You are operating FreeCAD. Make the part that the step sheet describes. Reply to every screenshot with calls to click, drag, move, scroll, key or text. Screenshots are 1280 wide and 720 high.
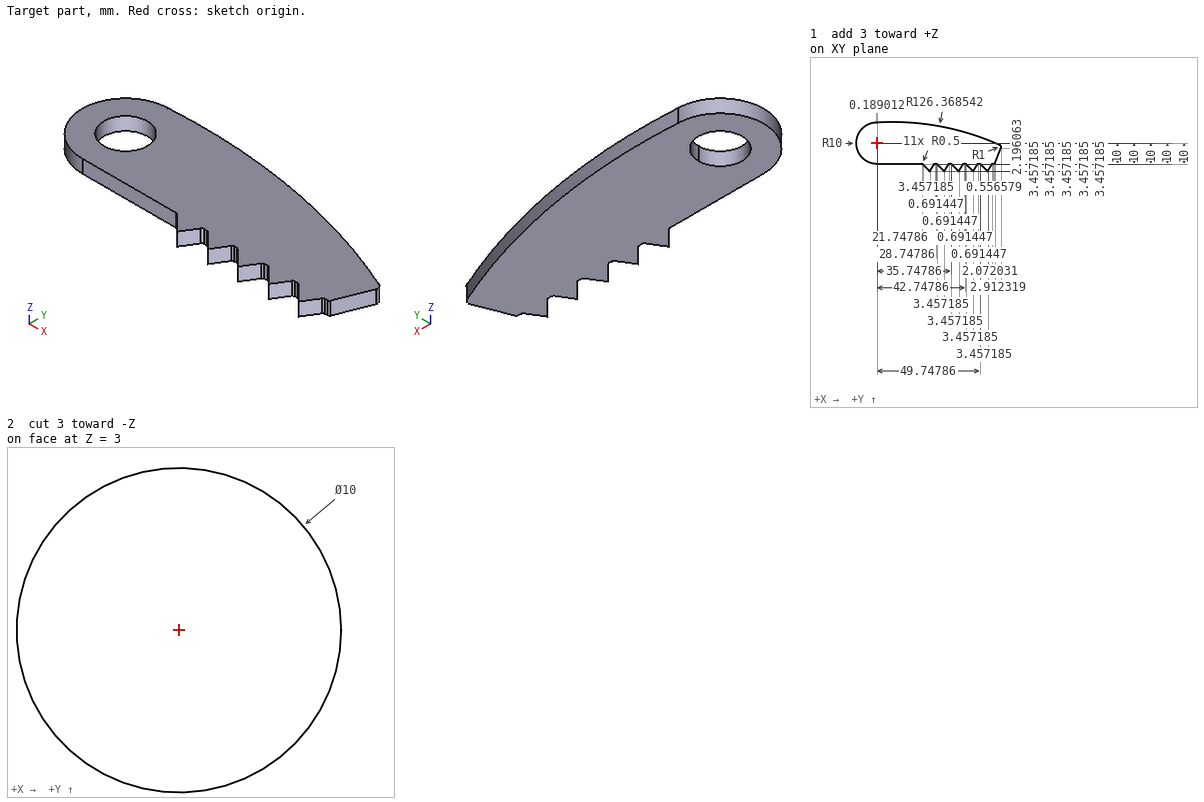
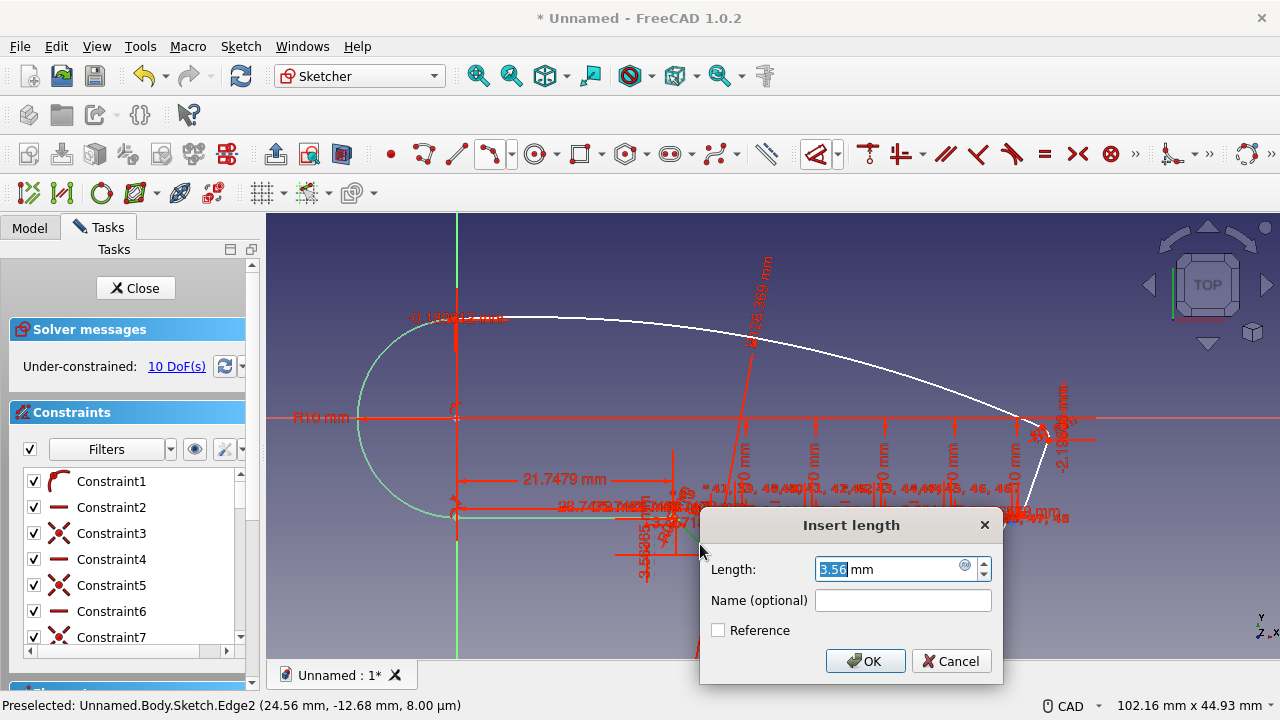
text(3.457185)
key(Return)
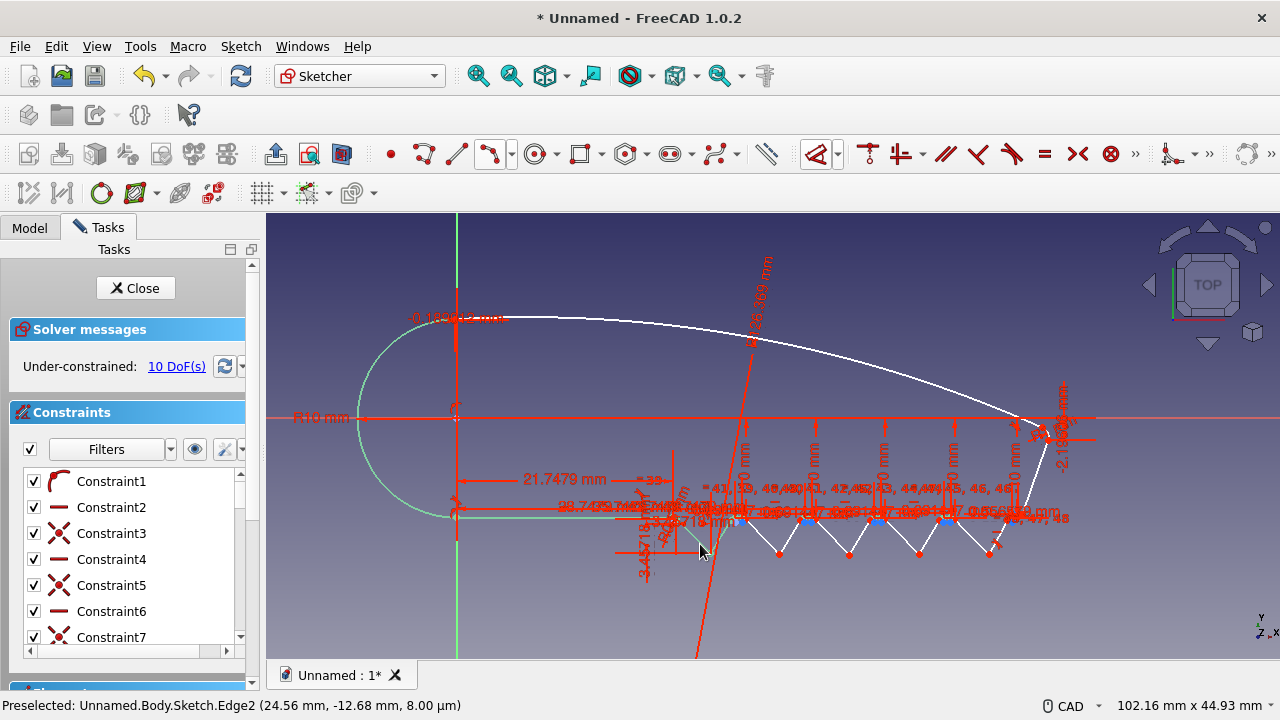
click(756, 530)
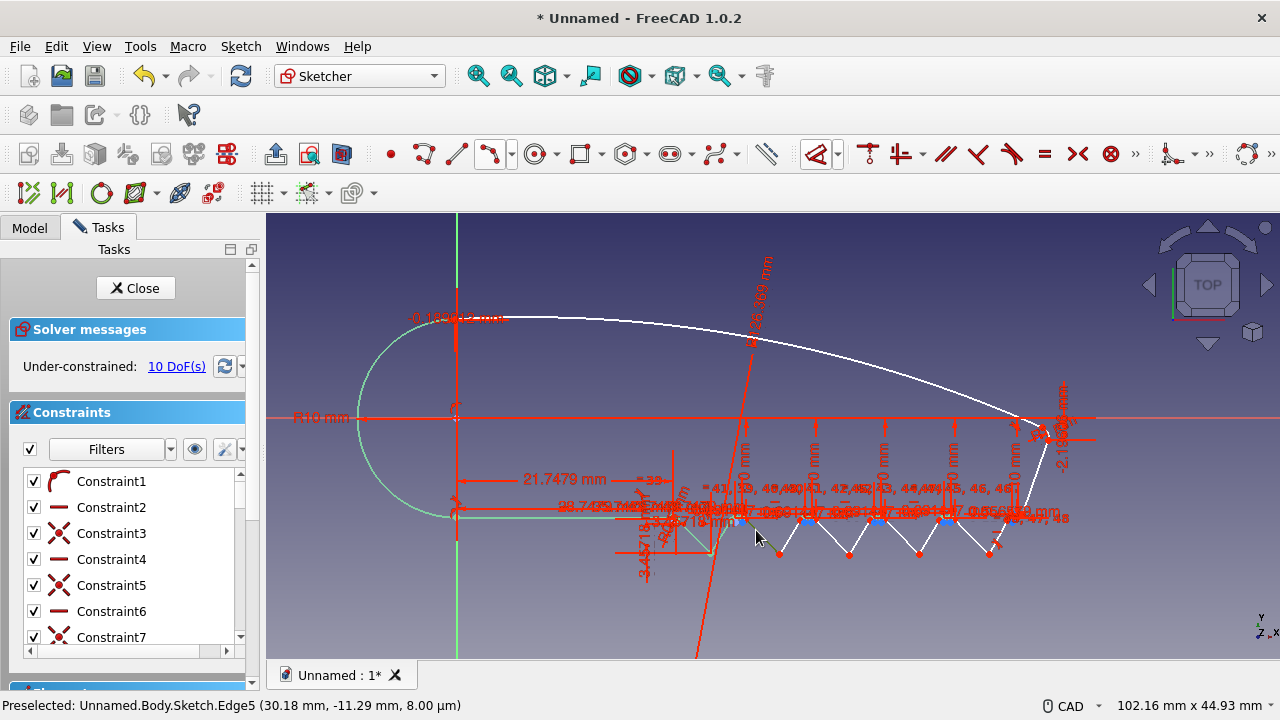
click(838, 154)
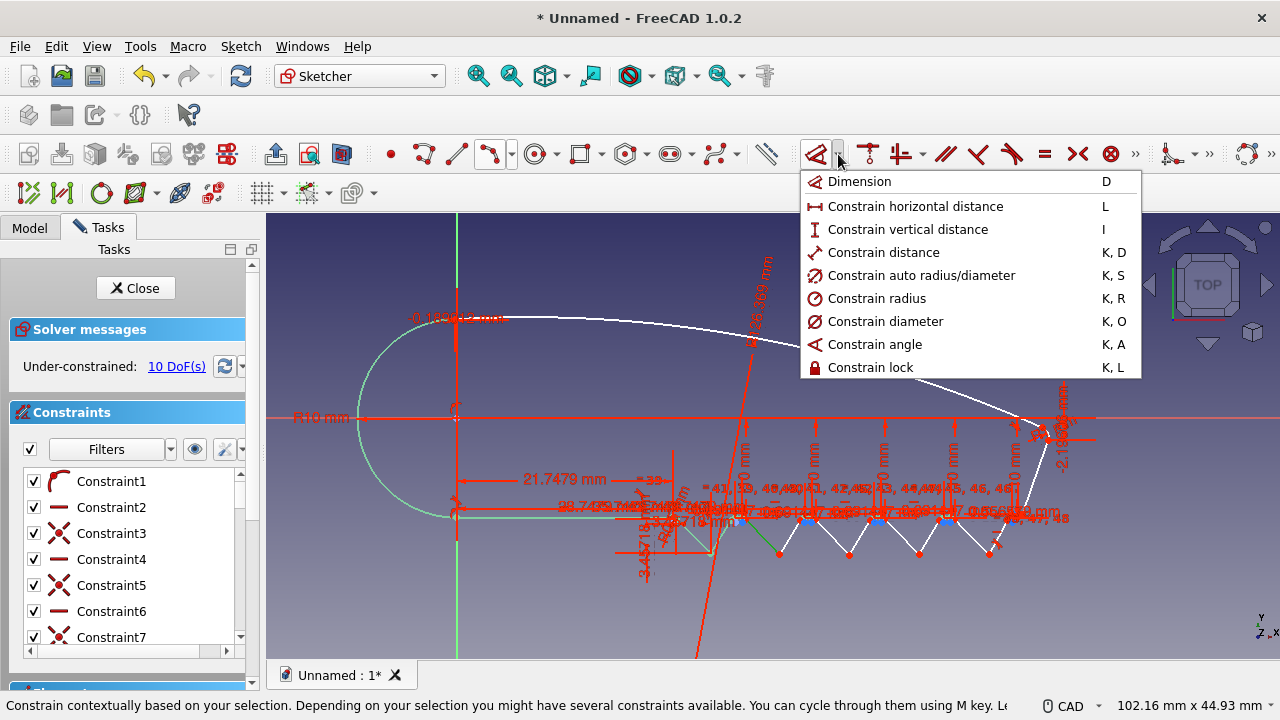
click(971, 206)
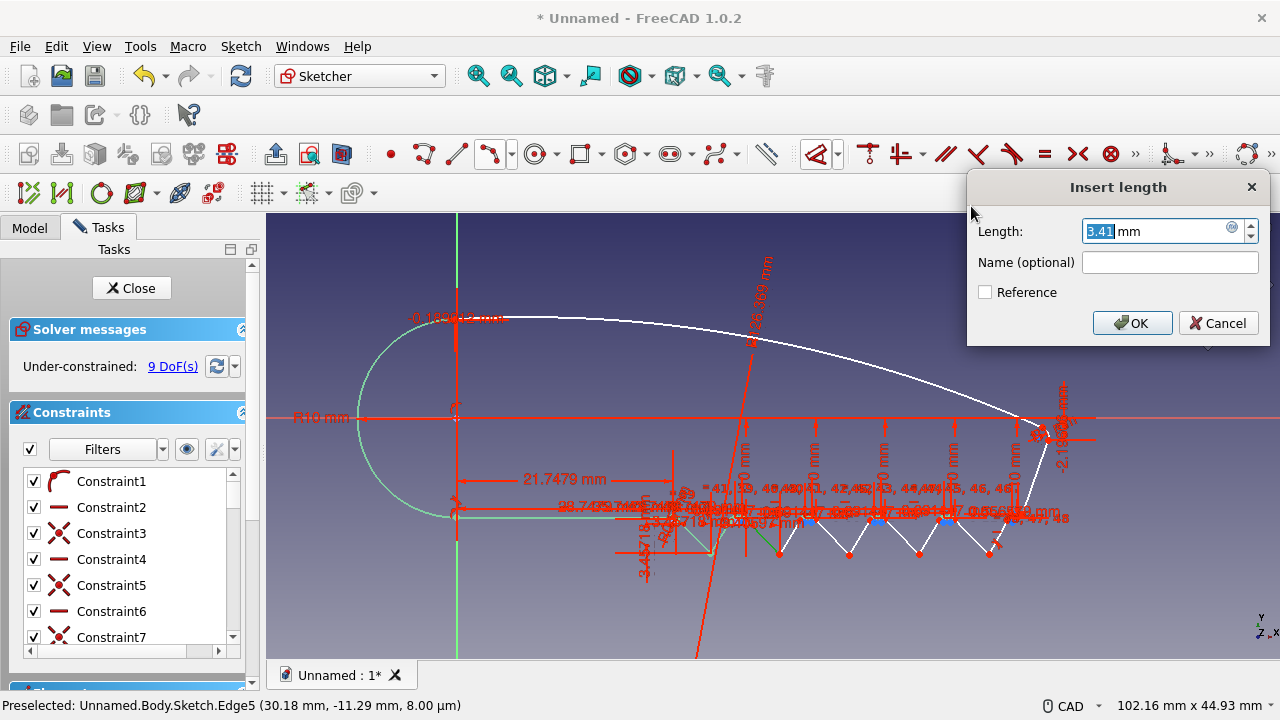
text(3.457185)
key(Return)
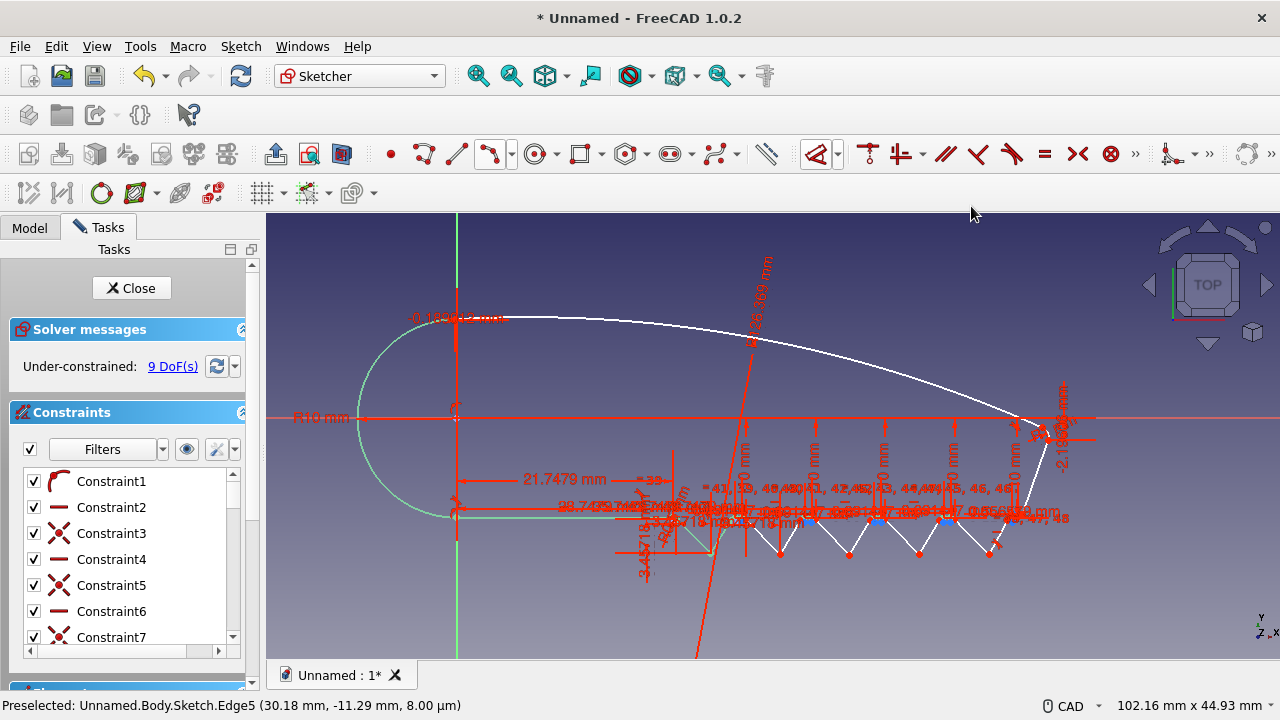
click(770, 544)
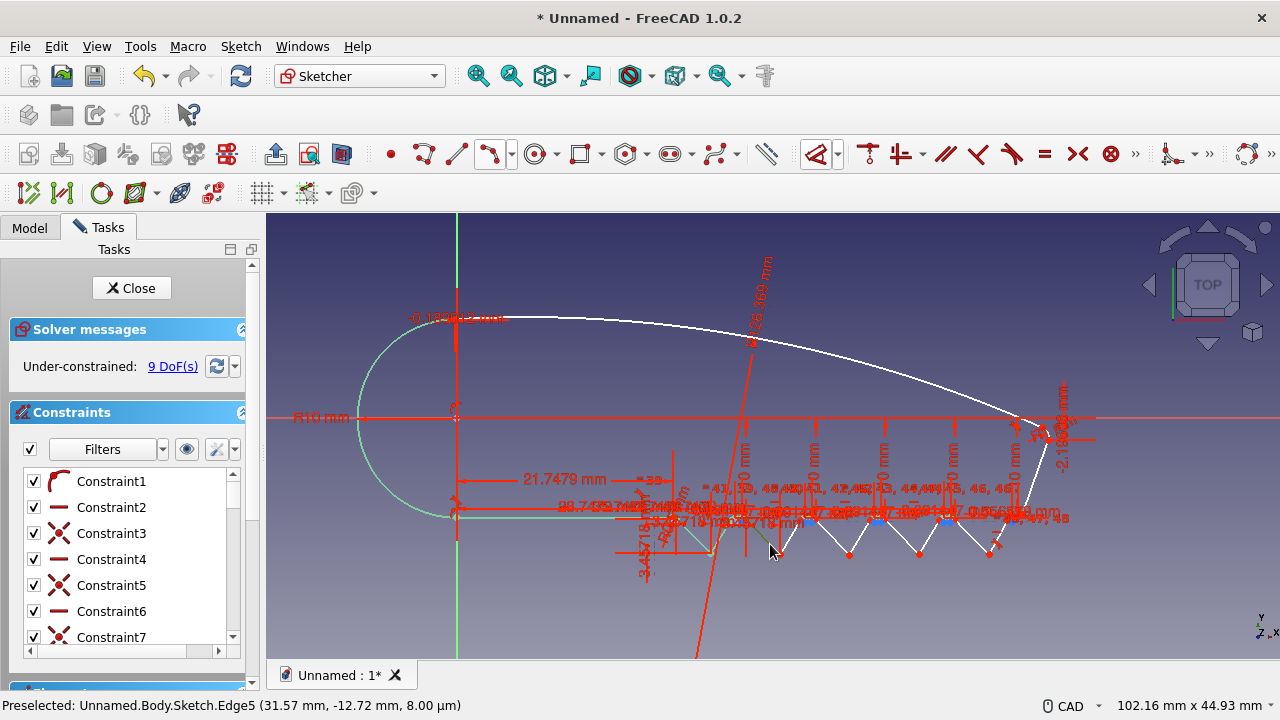
key(i)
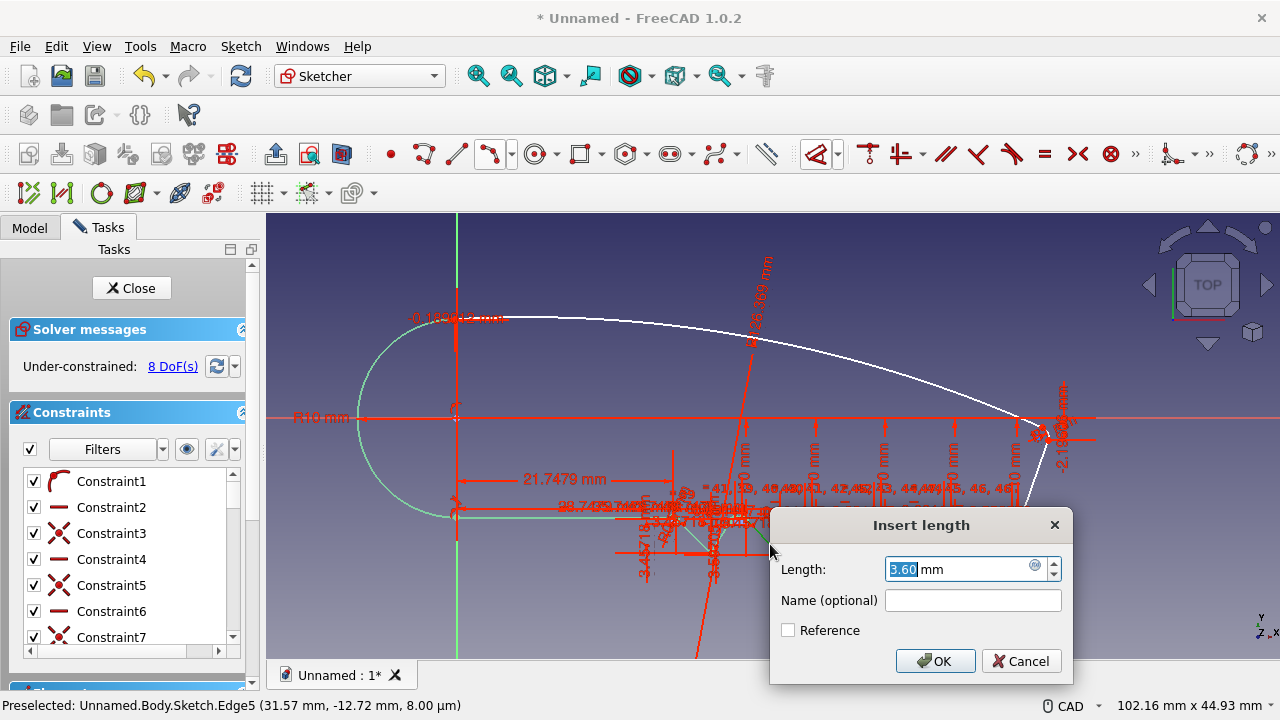
text(3.457185)
key(Return)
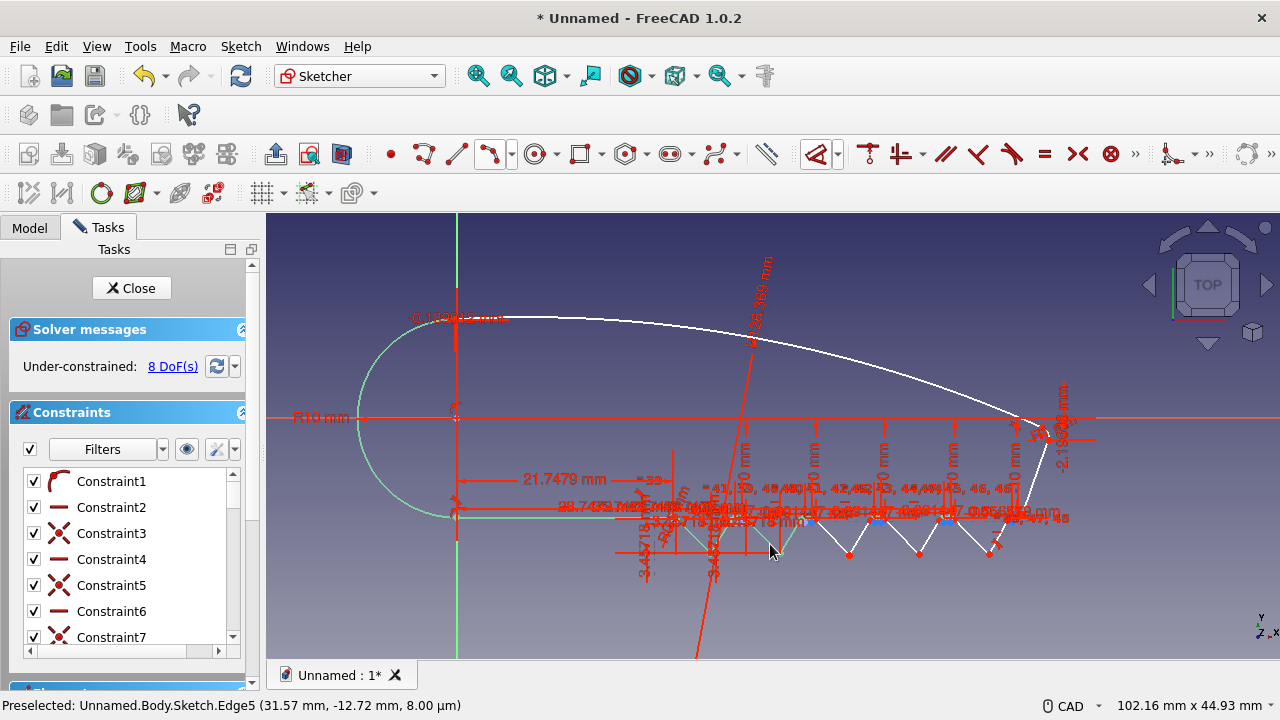
click(826, 530)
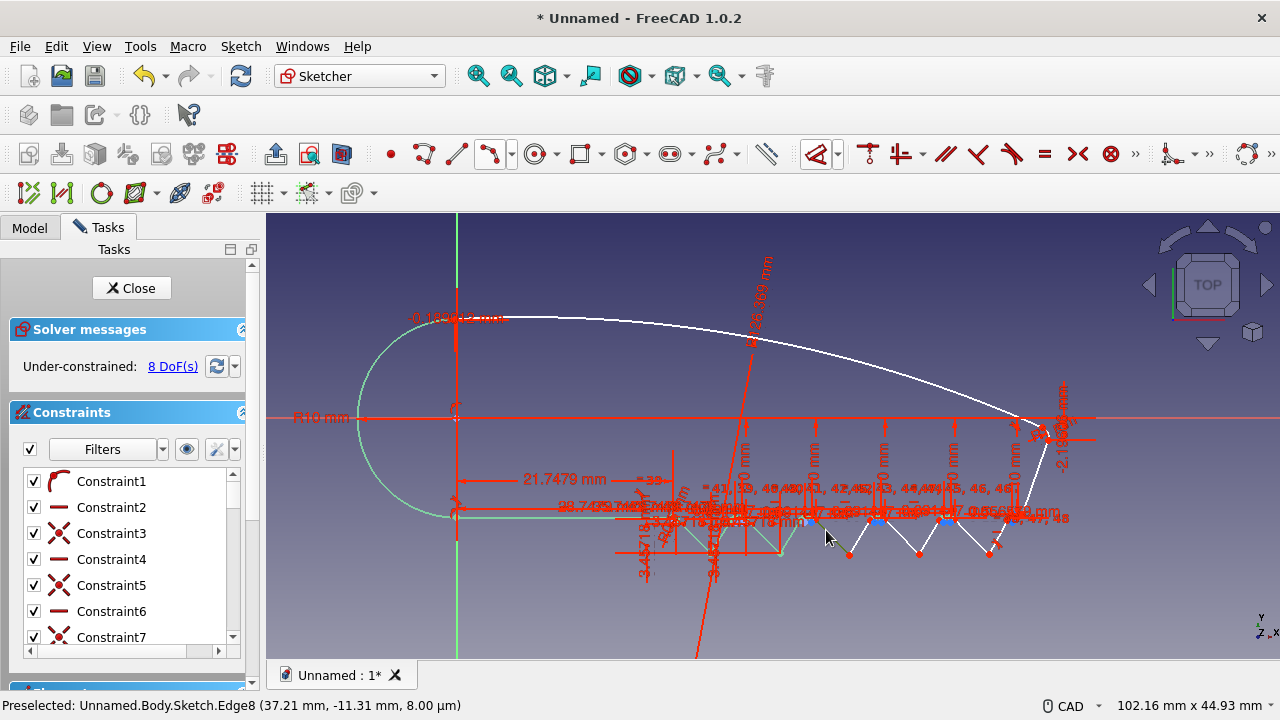
key(l)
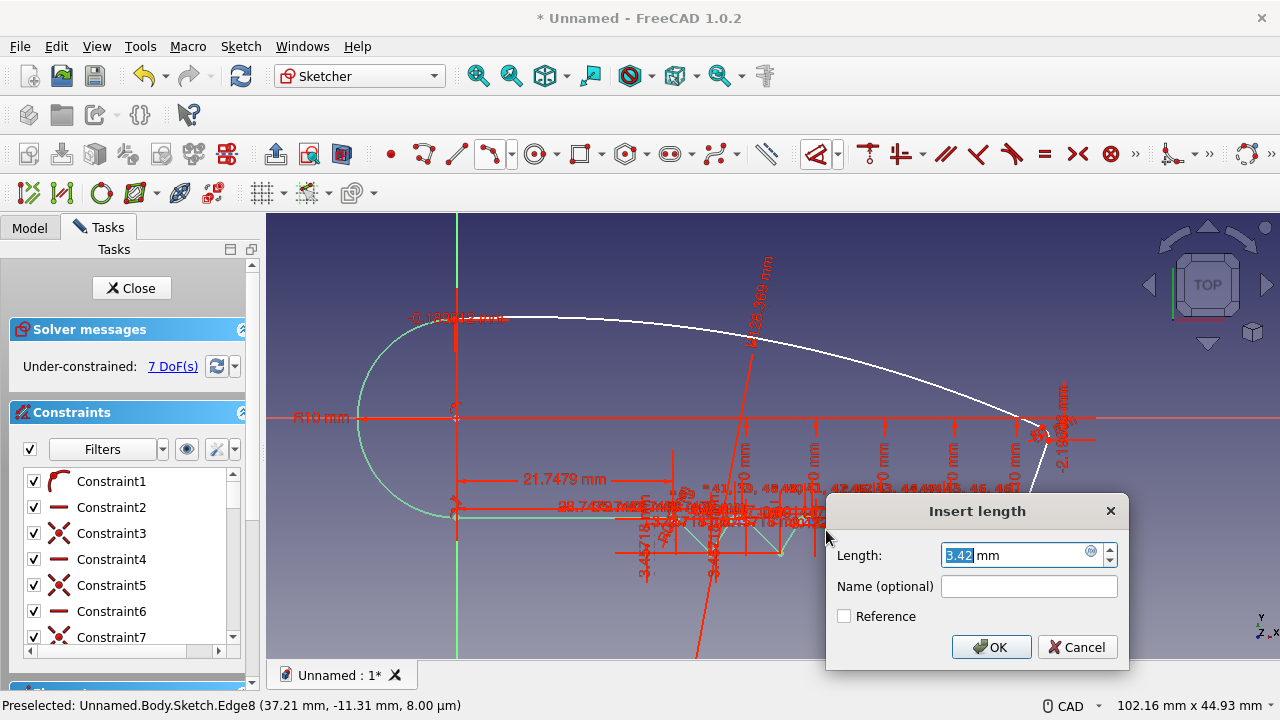
text(3.457185)
key(Return)